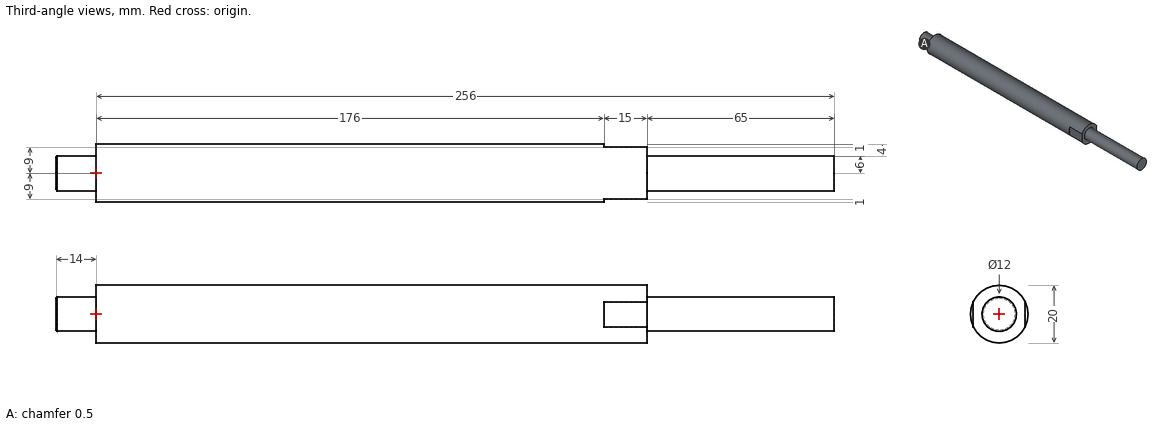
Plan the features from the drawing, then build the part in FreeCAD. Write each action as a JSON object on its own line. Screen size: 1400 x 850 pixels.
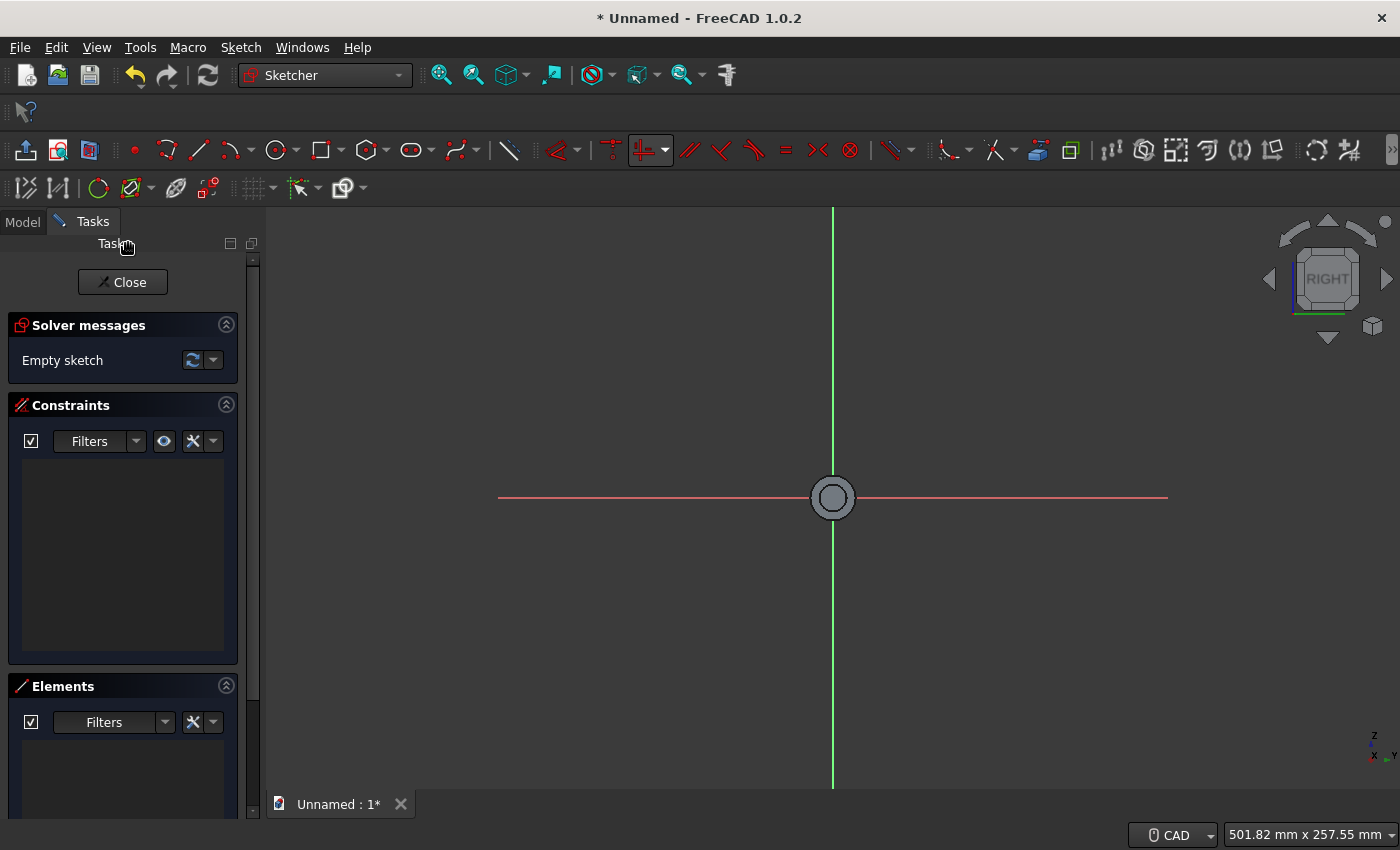
{"action": "key", "text": "q s"}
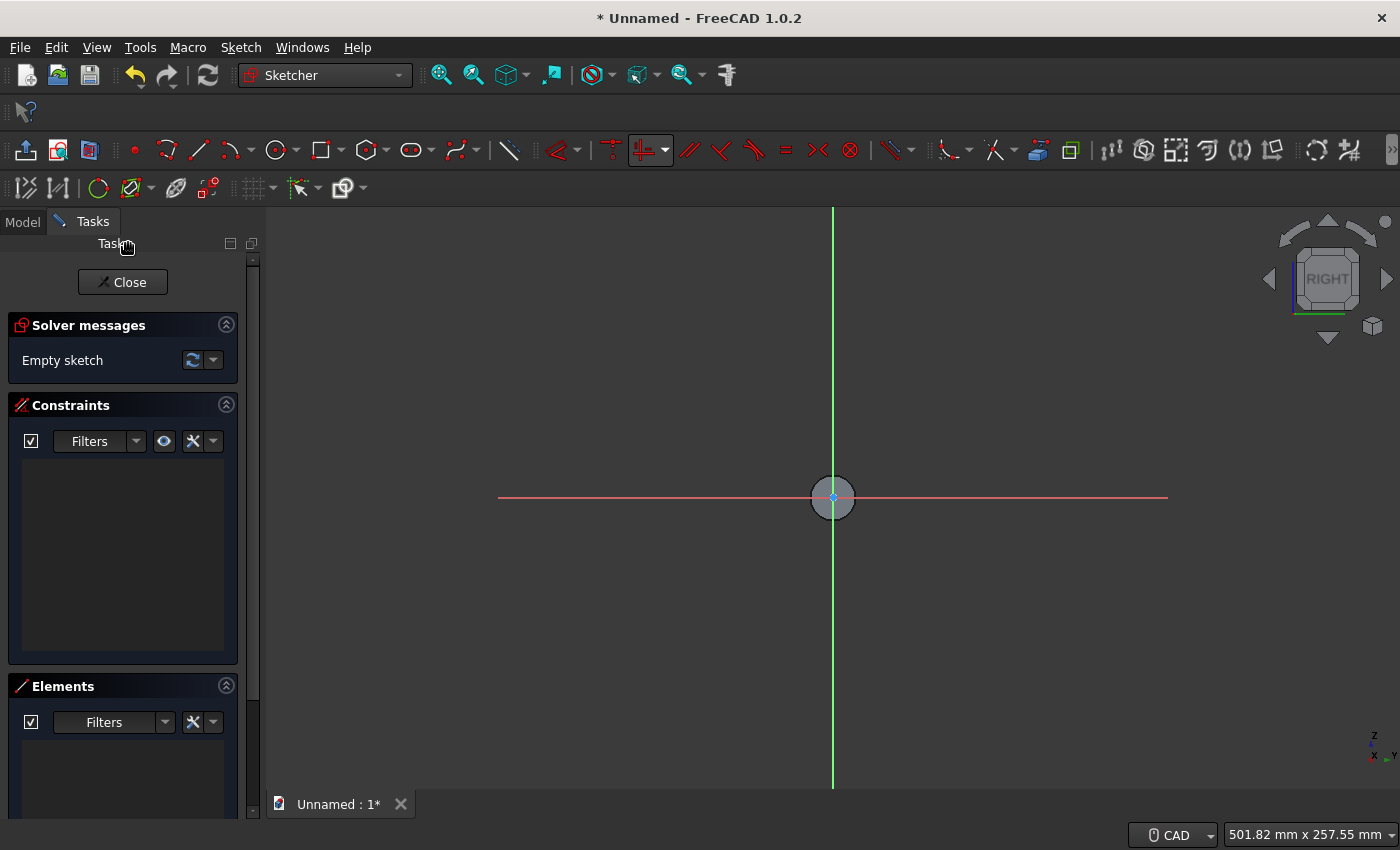
{"action": "scroll", "coordinate": [838, 498], "scroll_direction": "up", "scroll_amount": 13}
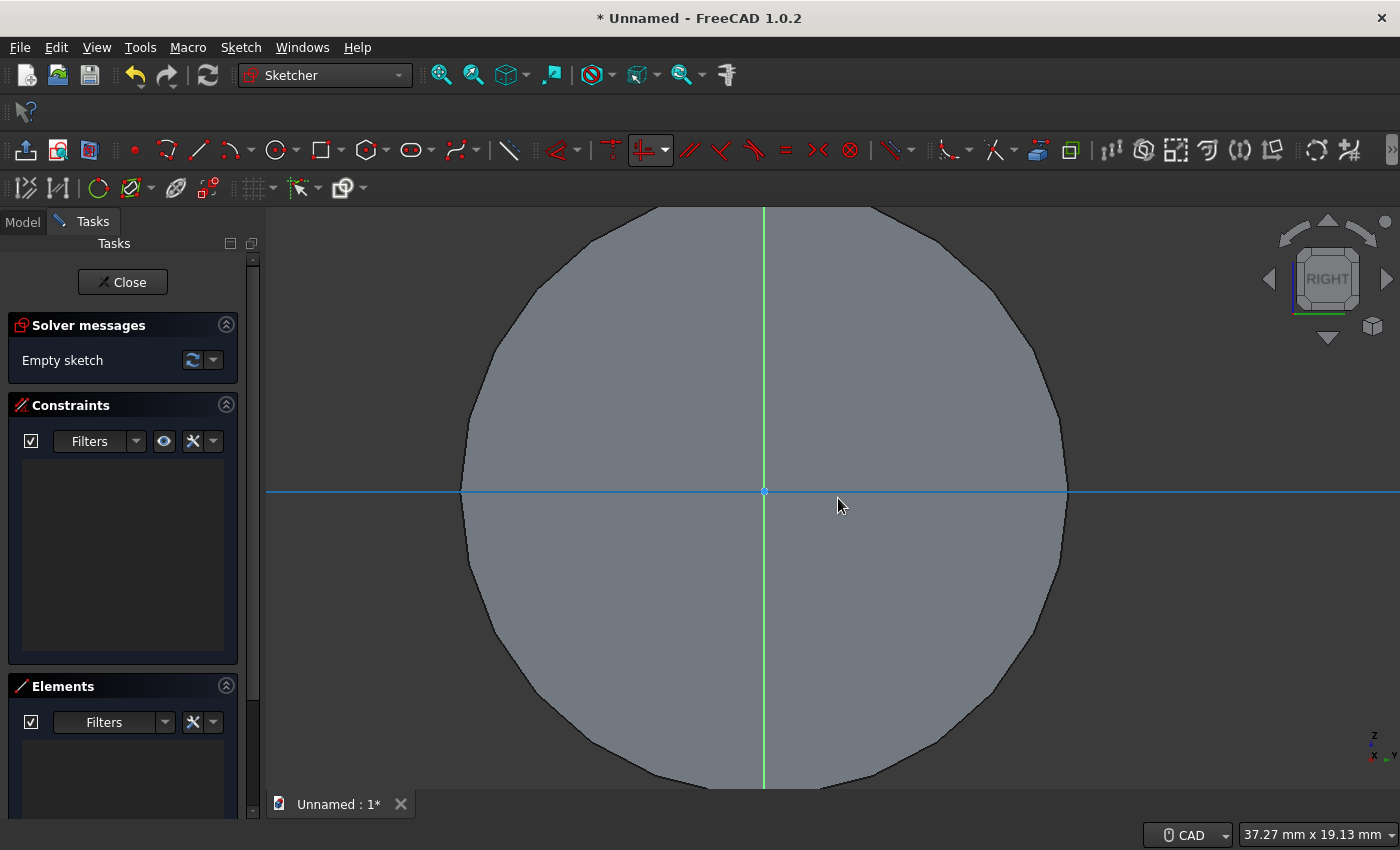
{"action": "key", "text": "g c"}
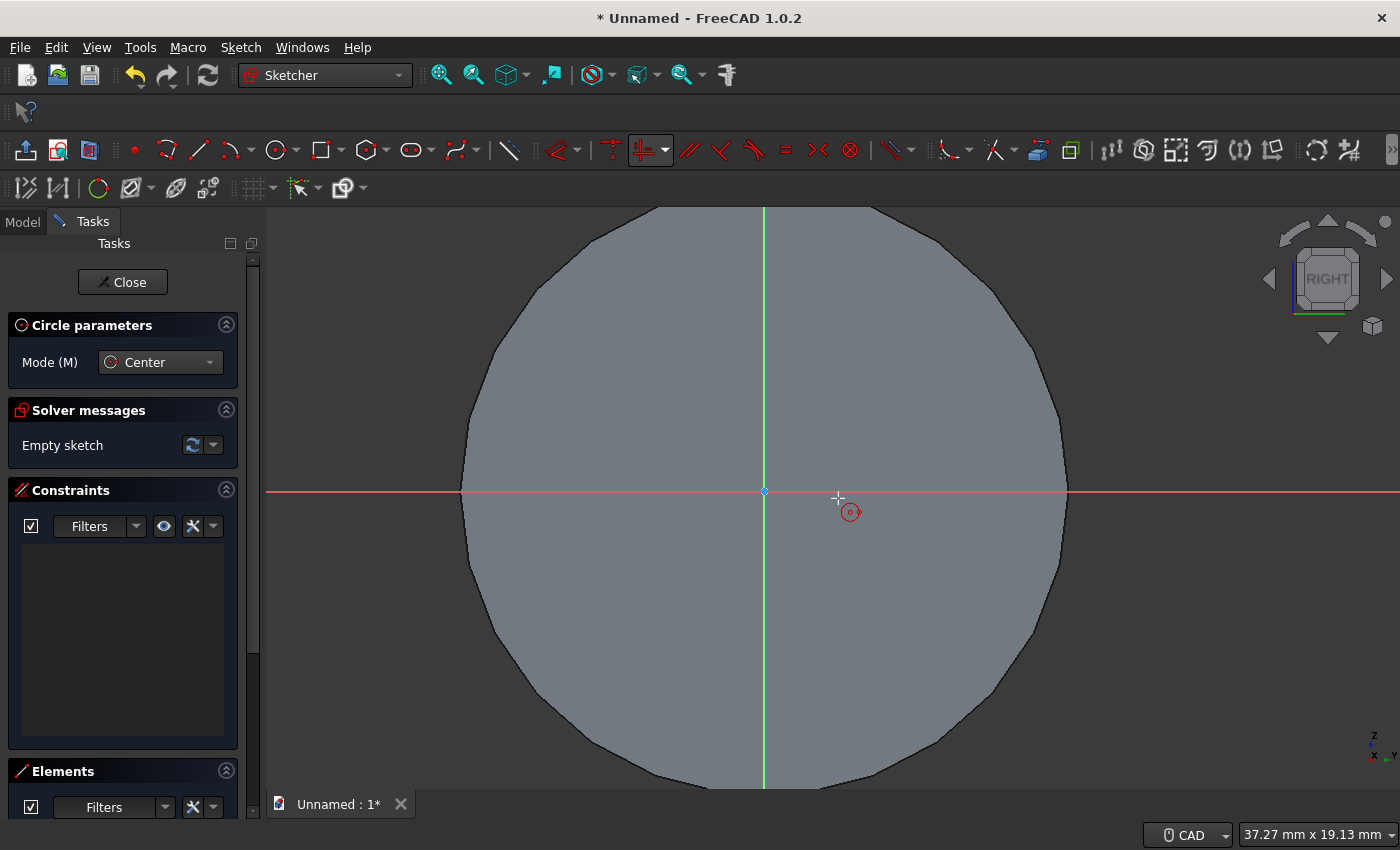
{"action": "left_click", "coordinate": [764, 492]}
{"action": "mouse_move", "coordinate": [893, 363]}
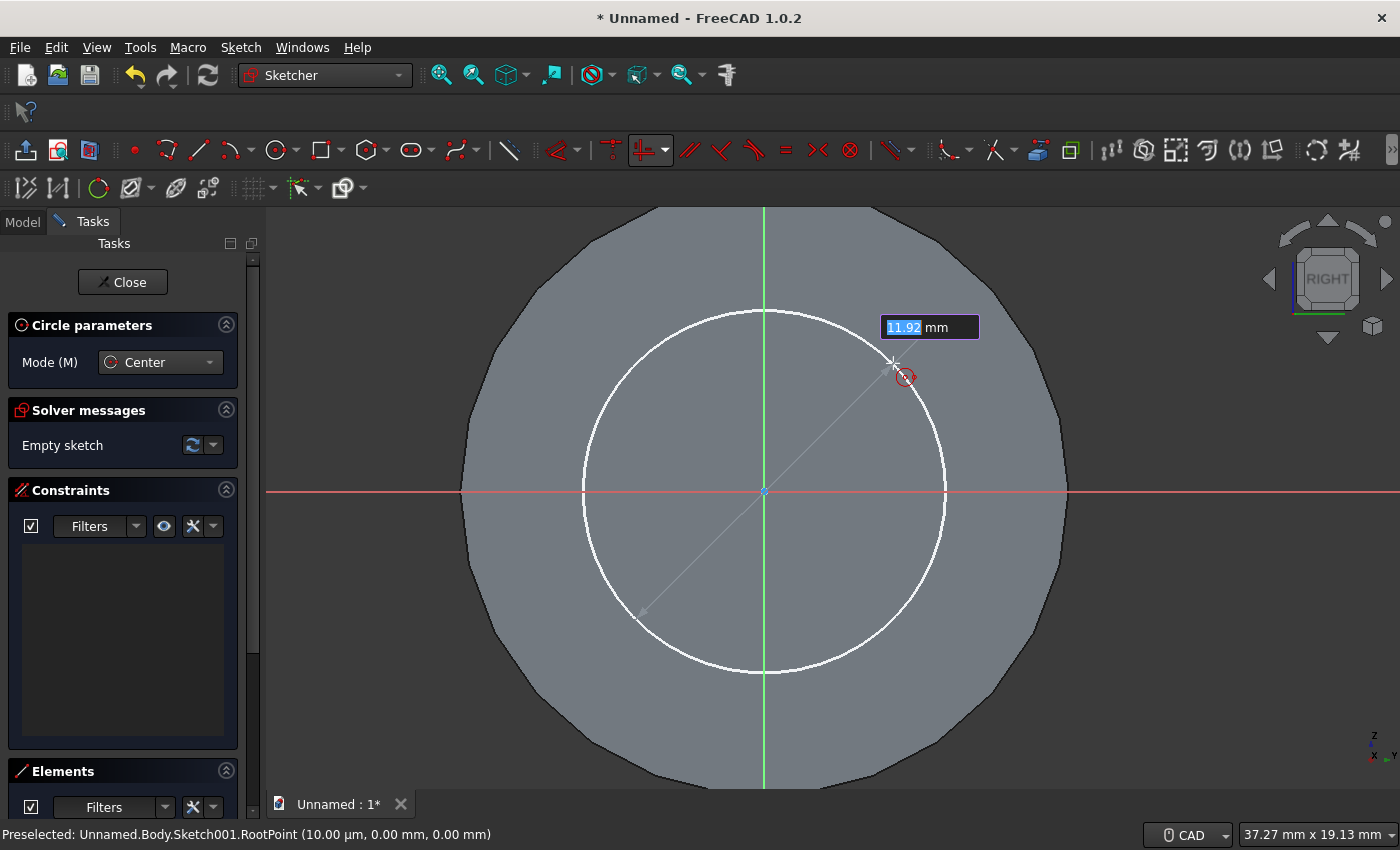
{"action": "type", "text": "12"}
{"action": "key", "text": "Return"}
{"action": "key", "text": "Escape"}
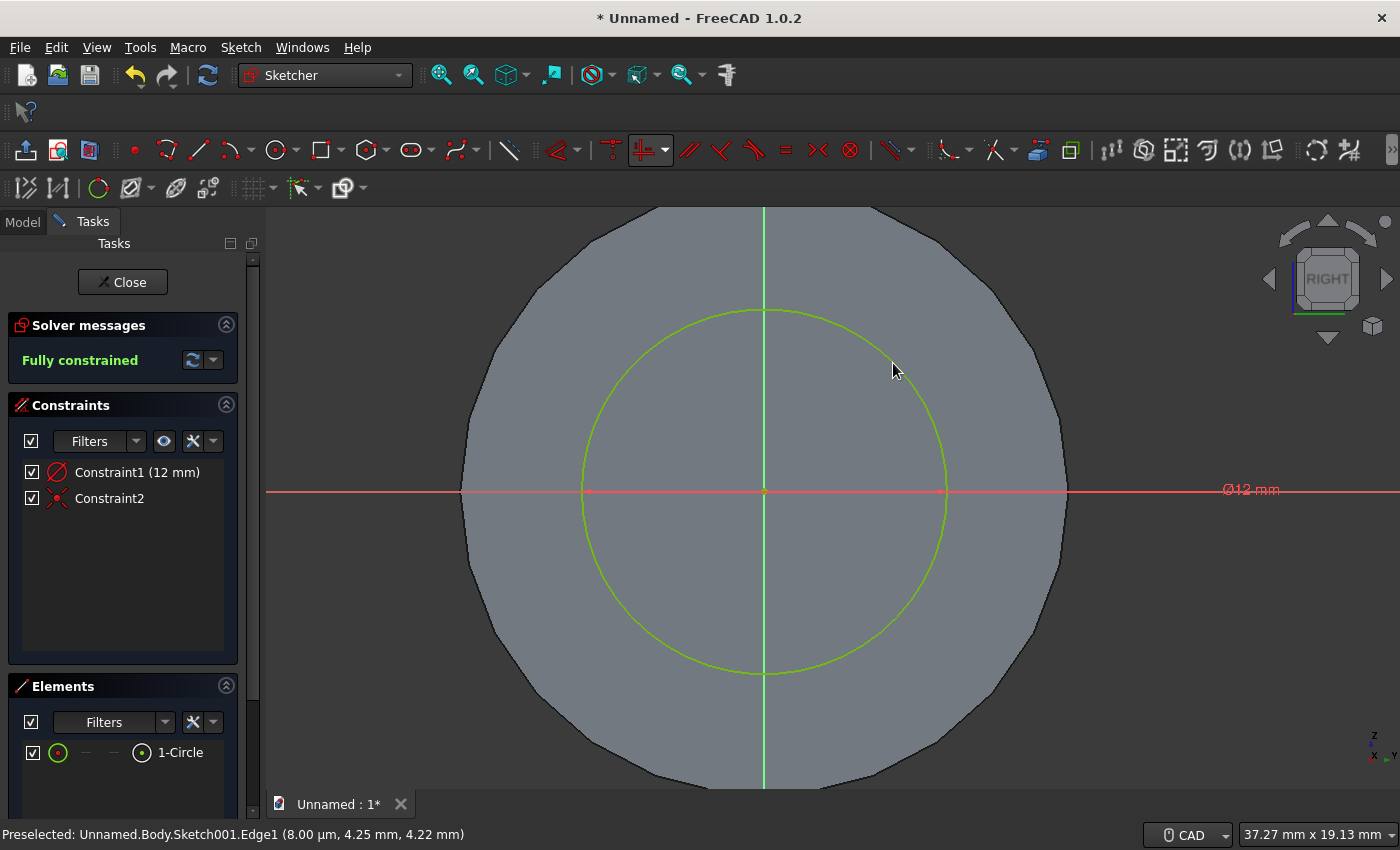
{"action": "left_click", "coordinate": [123, 282]}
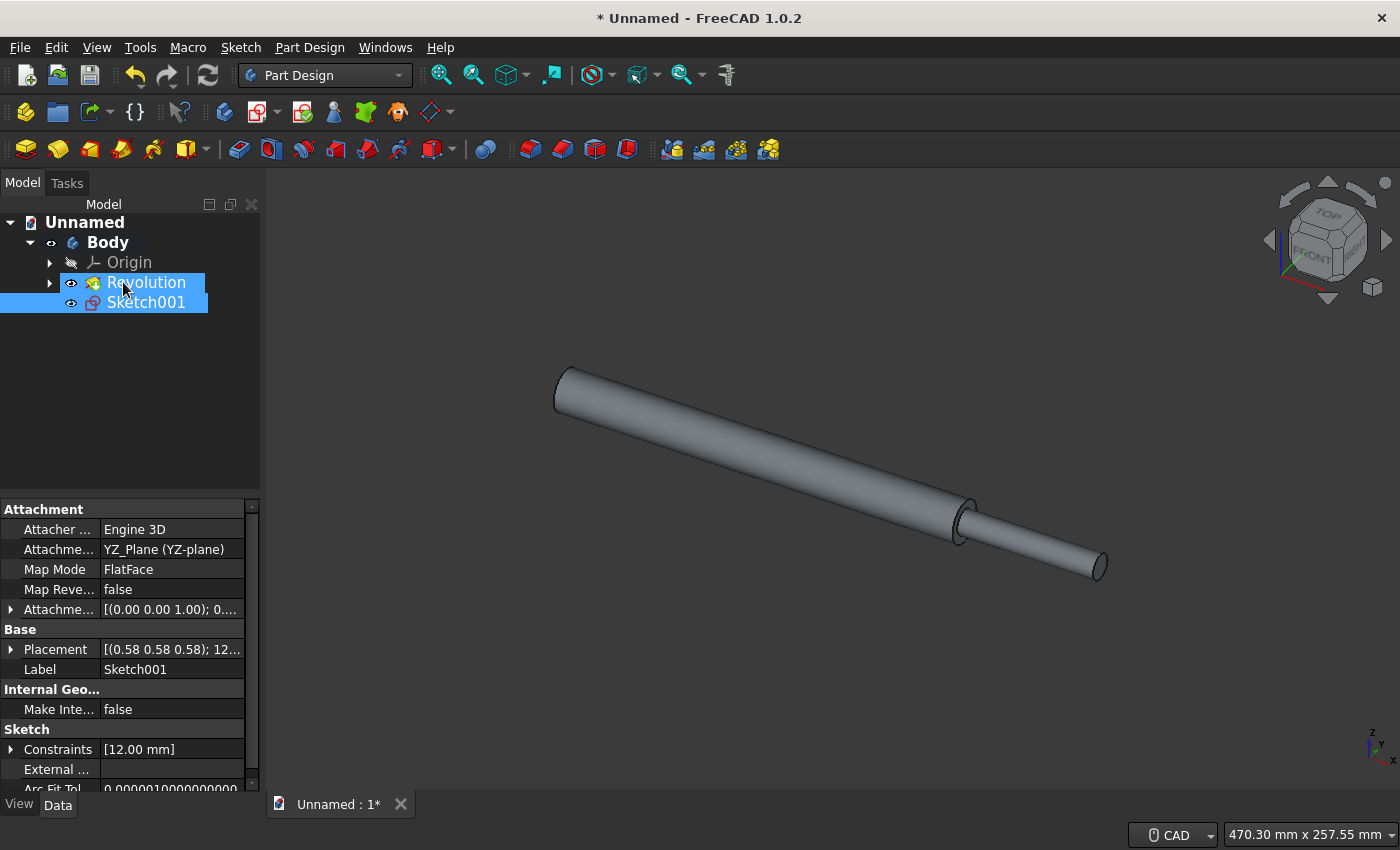
{"action": "left_click", "coordinate": [26, 150]}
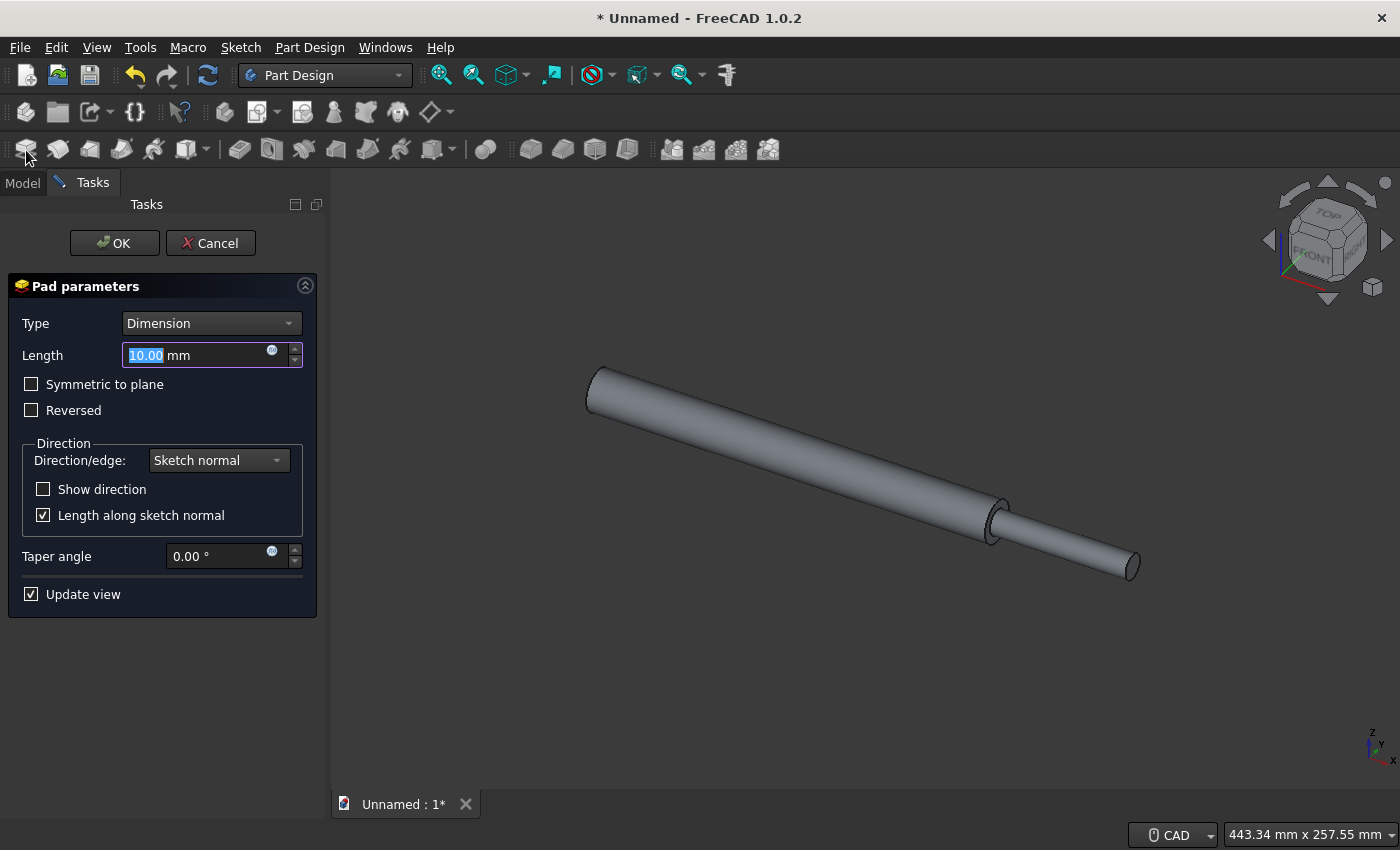
{"action": "type", "text": "14"}
{"action": "key", "text": "Tab"}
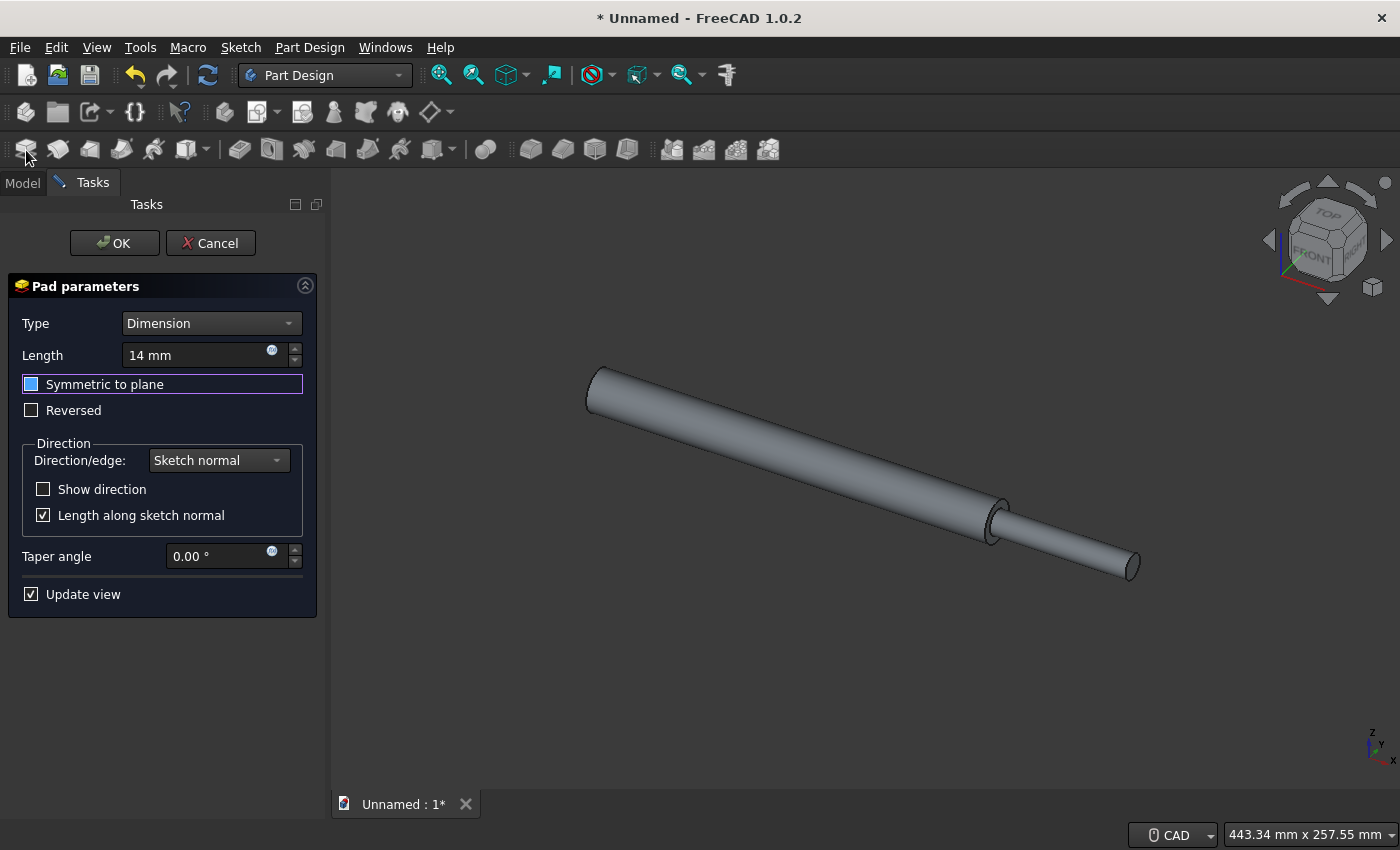
{"action": "left_click", "coordinate": [30, 410]}